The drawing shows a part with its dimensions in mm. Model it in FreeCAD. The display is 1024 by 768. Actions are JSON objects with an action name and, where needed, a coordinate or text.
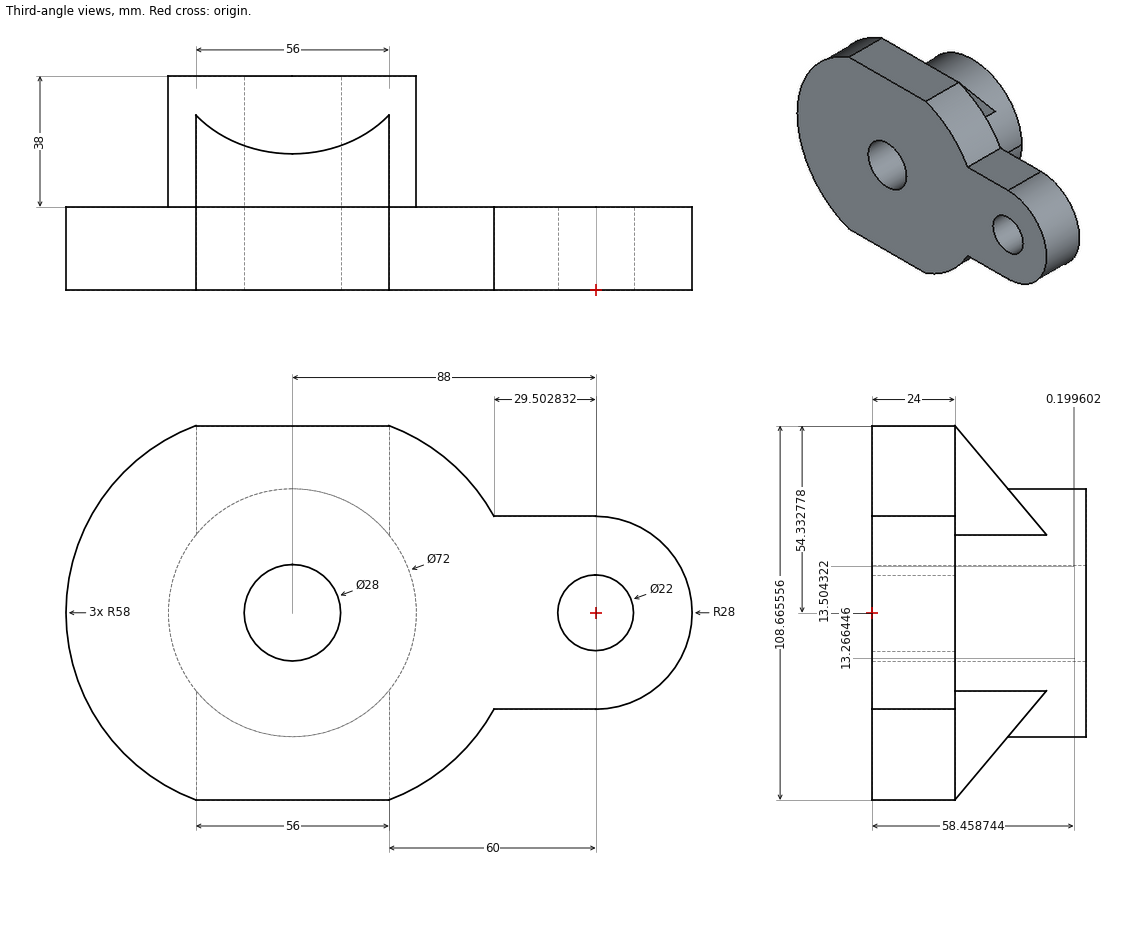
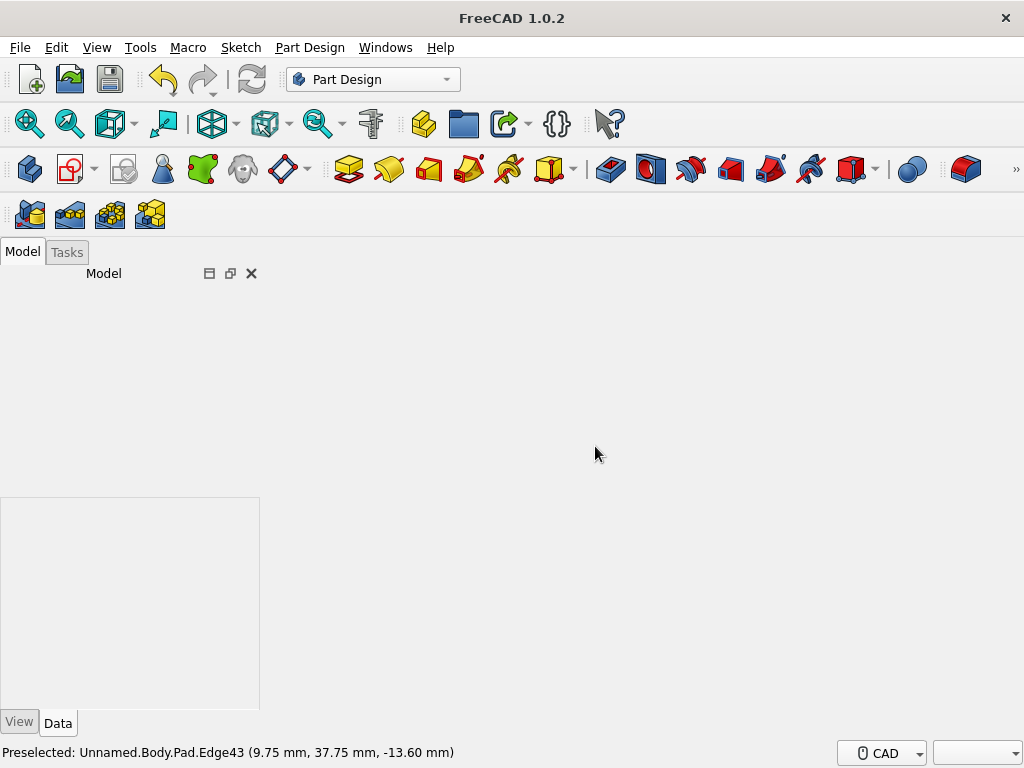
{"action": "key", "text": "ctrl+n"}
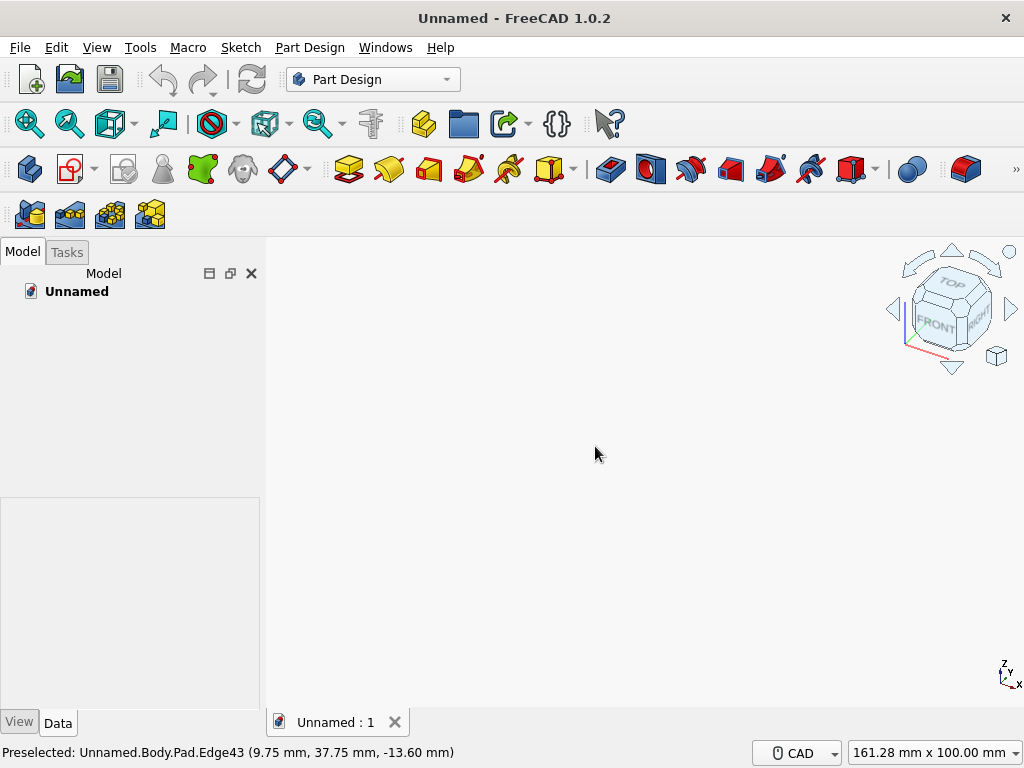
{"action": "left_click", "coordinate": [70, 170]}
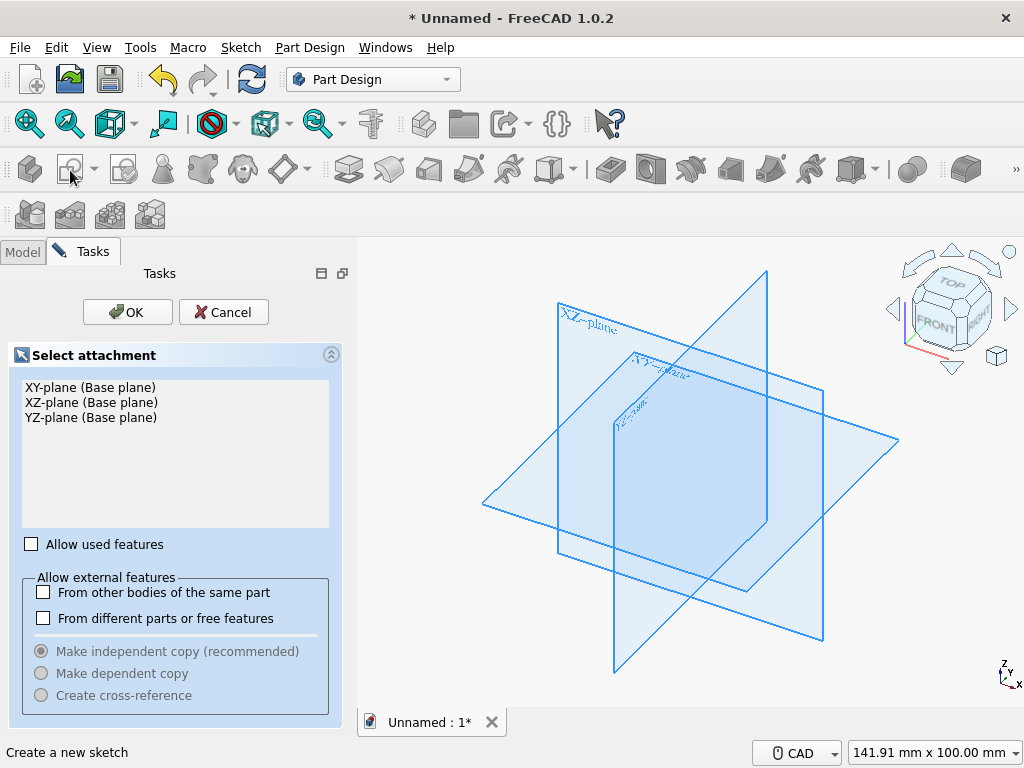
{"action": "left_click", "coordinate": [82, 402]}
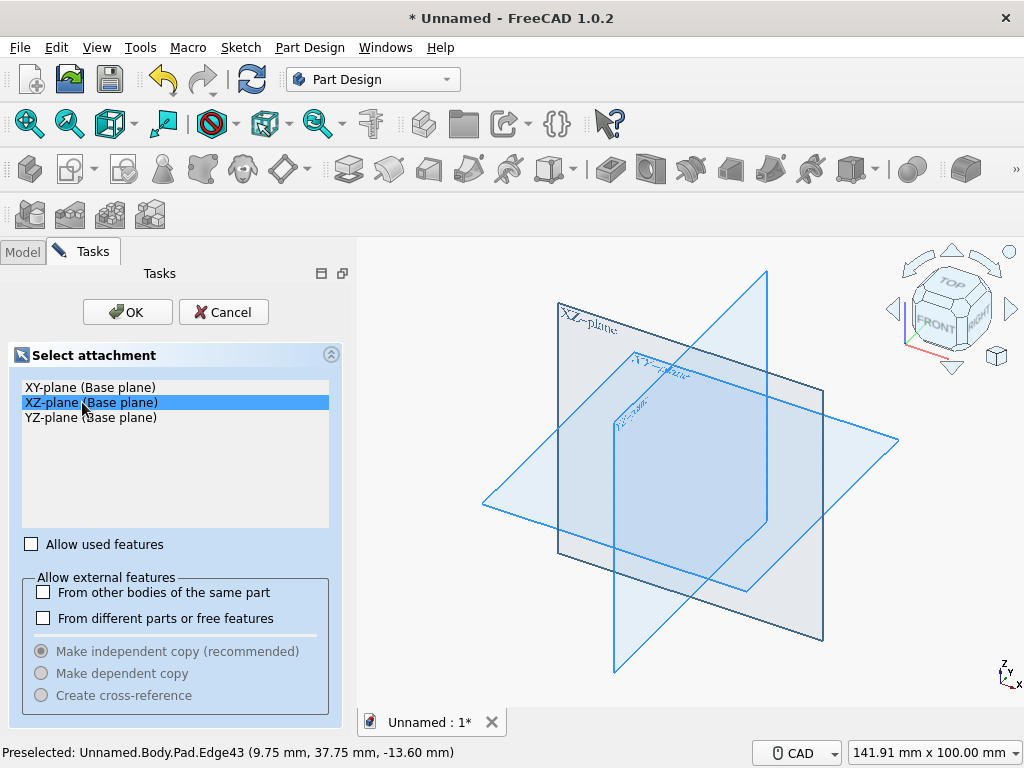
{"action": "left_click", "coordinate": [128, 312]}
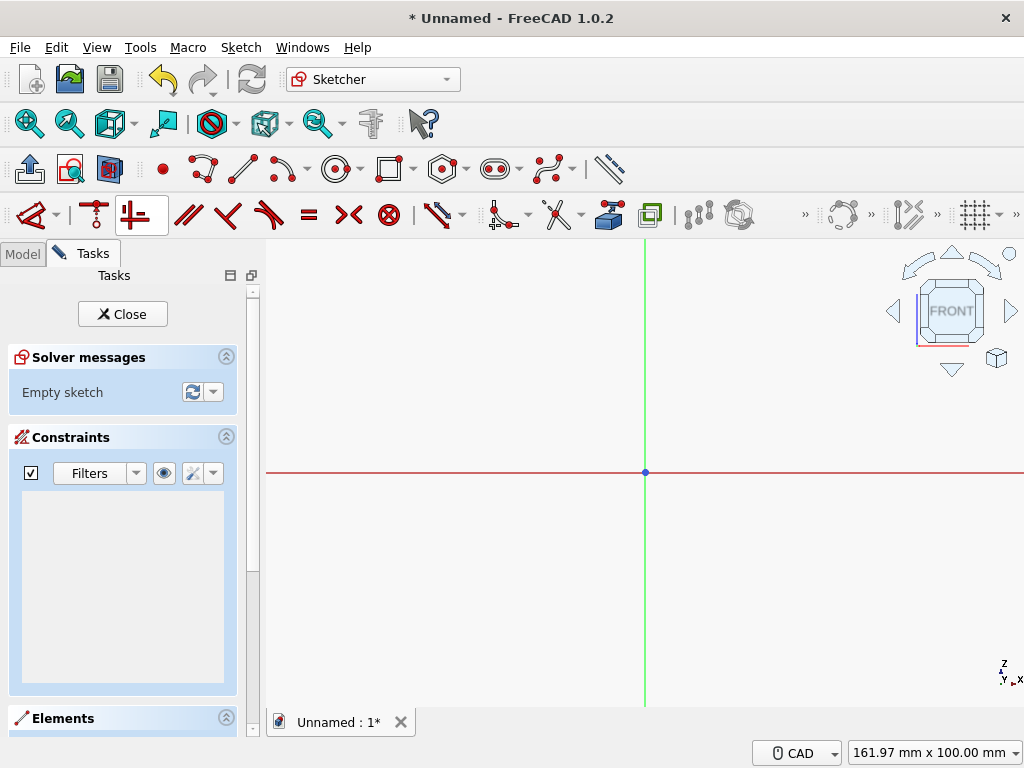
{"action": "scroll", "coordinate": [761, 473], "scroll_direction": "down", "scroll_amount": 4}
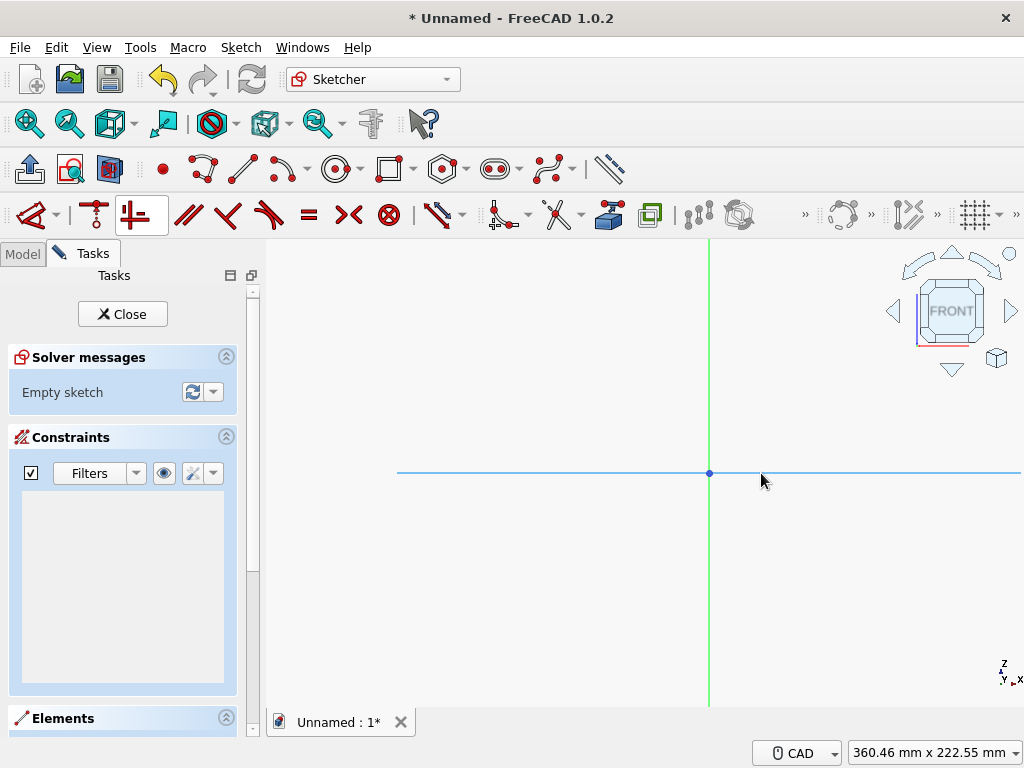
{"action": "left_click", "coordinate": [244, 170]}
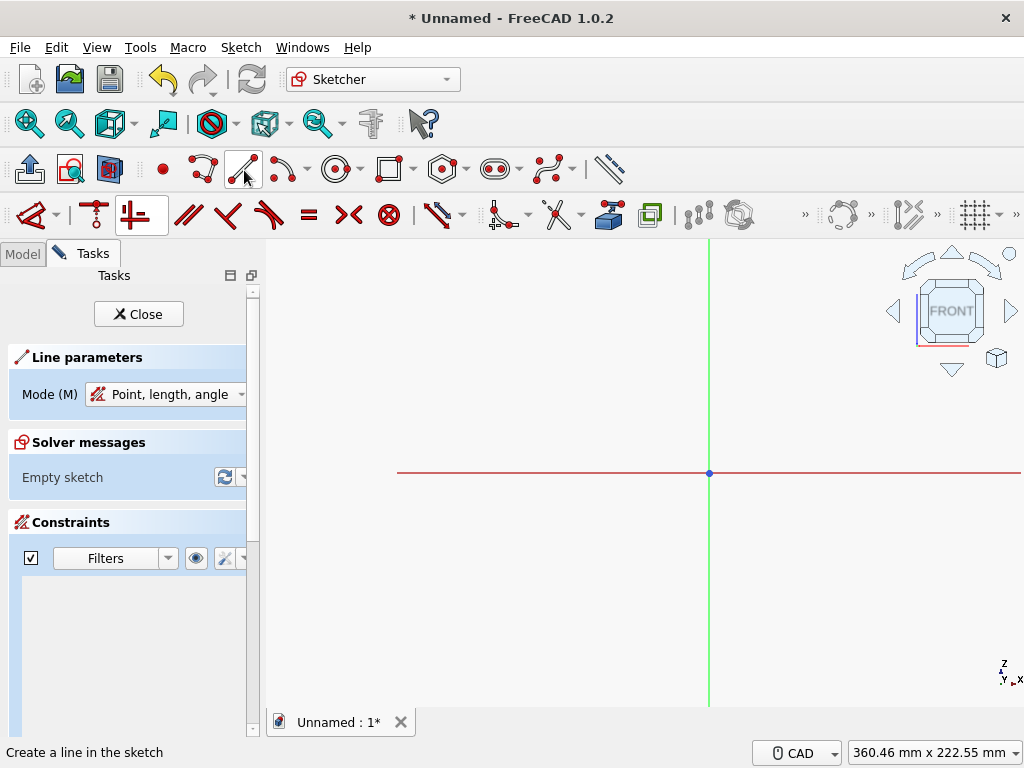
{"action": "left_click", "coordinate": [583, 588]}
{"action": "left_click", "coordinate": [465, 588]}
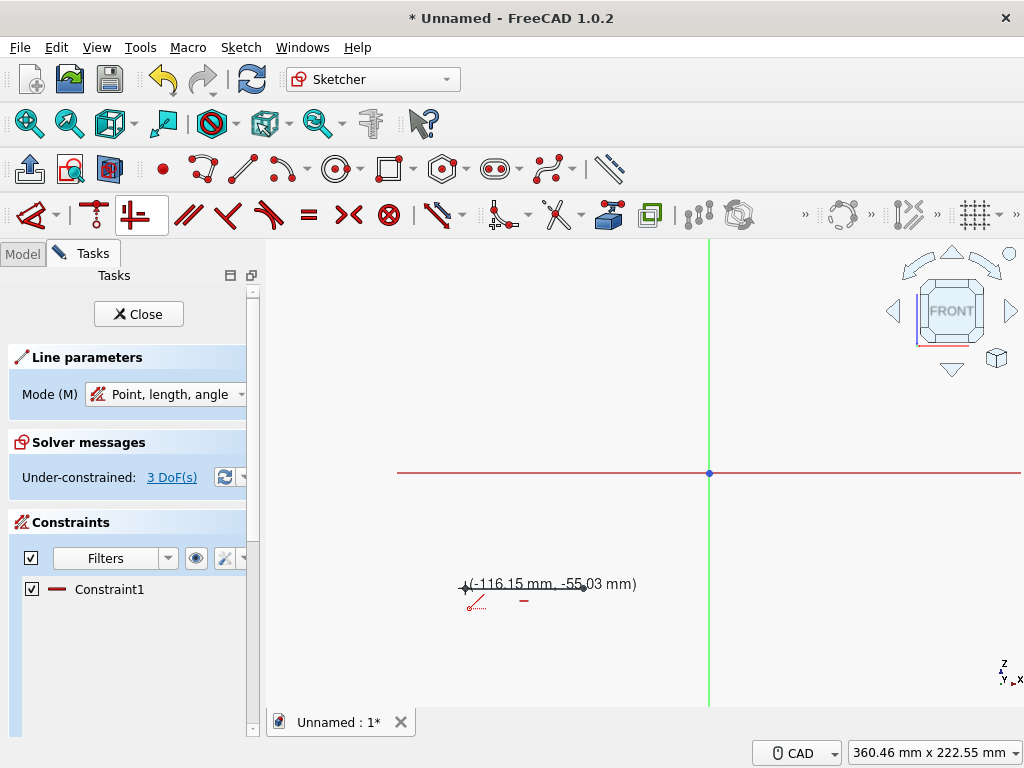
{"action": "left_click", "coordinate": [465, 359]}
{"action": "left_click", "coordinate": [583, 359]}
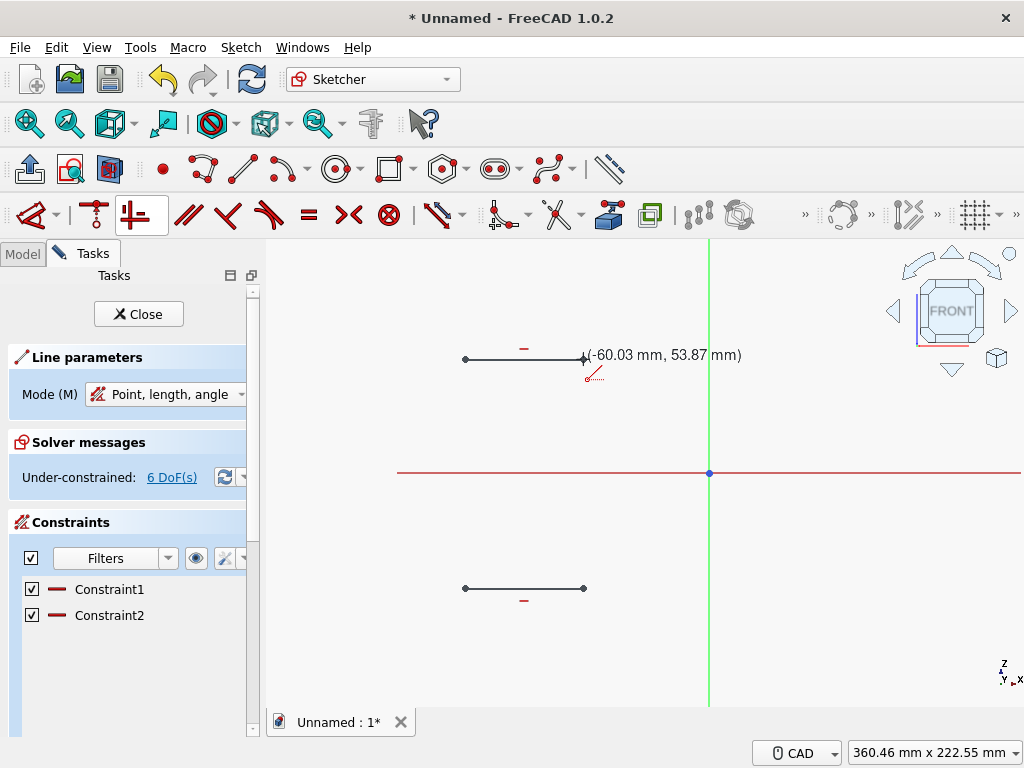
{"action": "left_click", "coordinate": [647, 414]}
{"action": "left_click", "coordinate": [709, 414]}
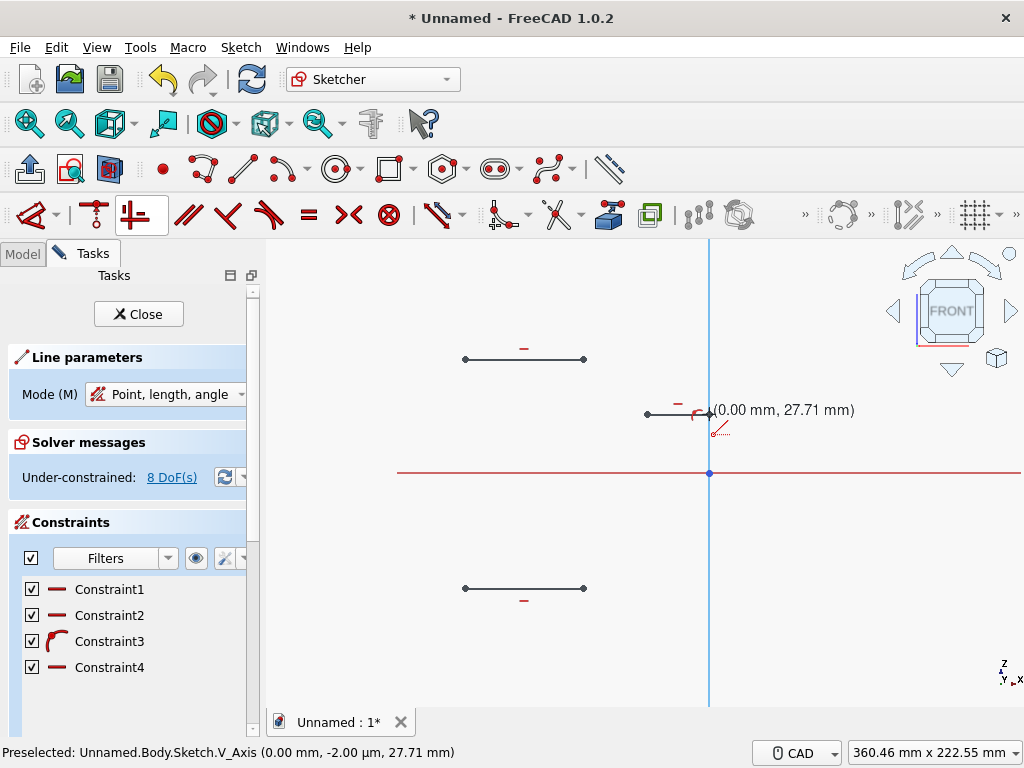
{"action": "left_click", "coordinate": [709, 532]}
{"action": "left_click", "coordinate": [647, 532]}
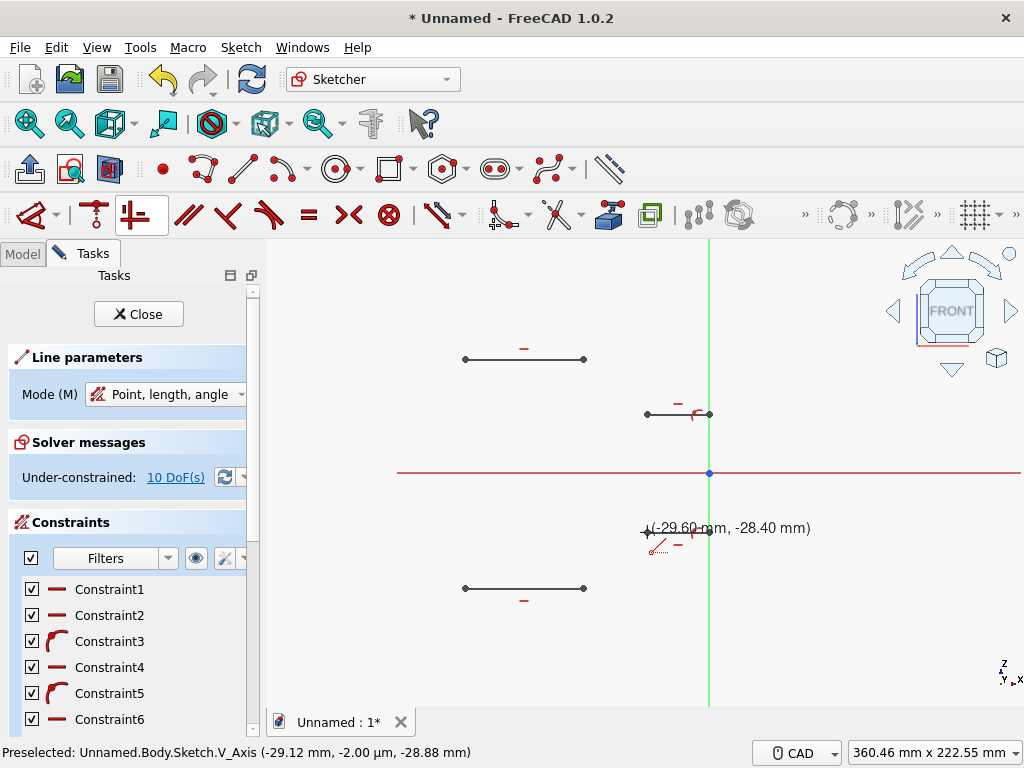
{"action": "key", "text": "g 3 a"}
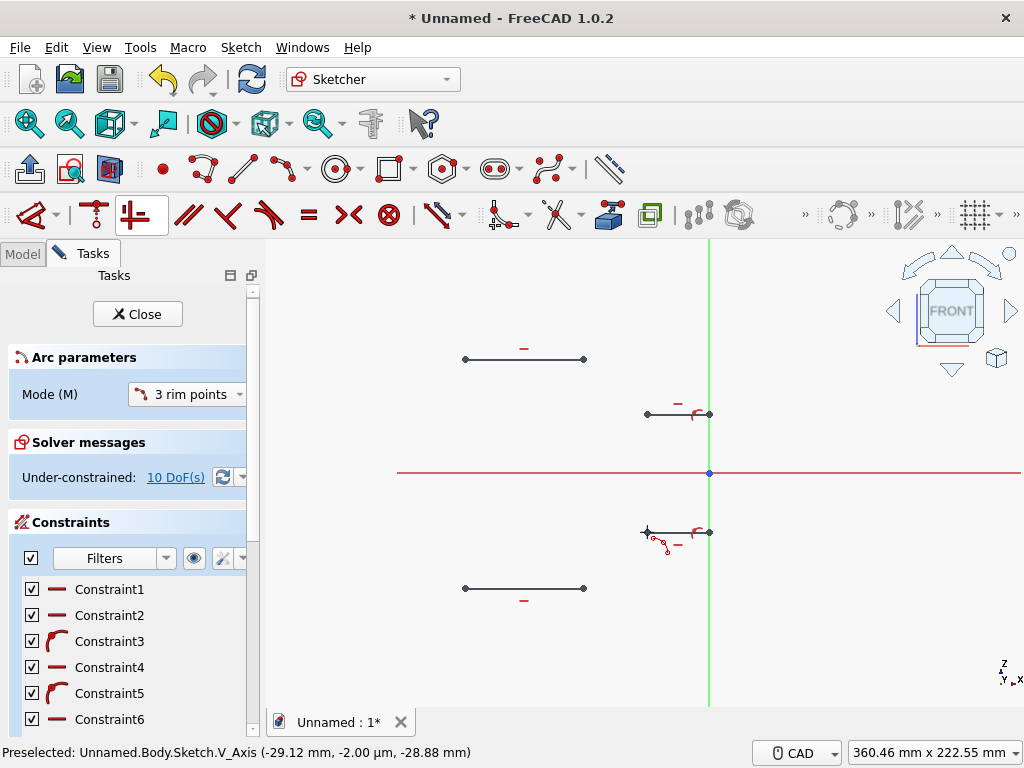
{"action": "left_click", "coordinate": [465, 589]}
{"action": "left_click", "coordinate": [465, 360]}
{"action": "left_click", "coordinate": [390, 444]}